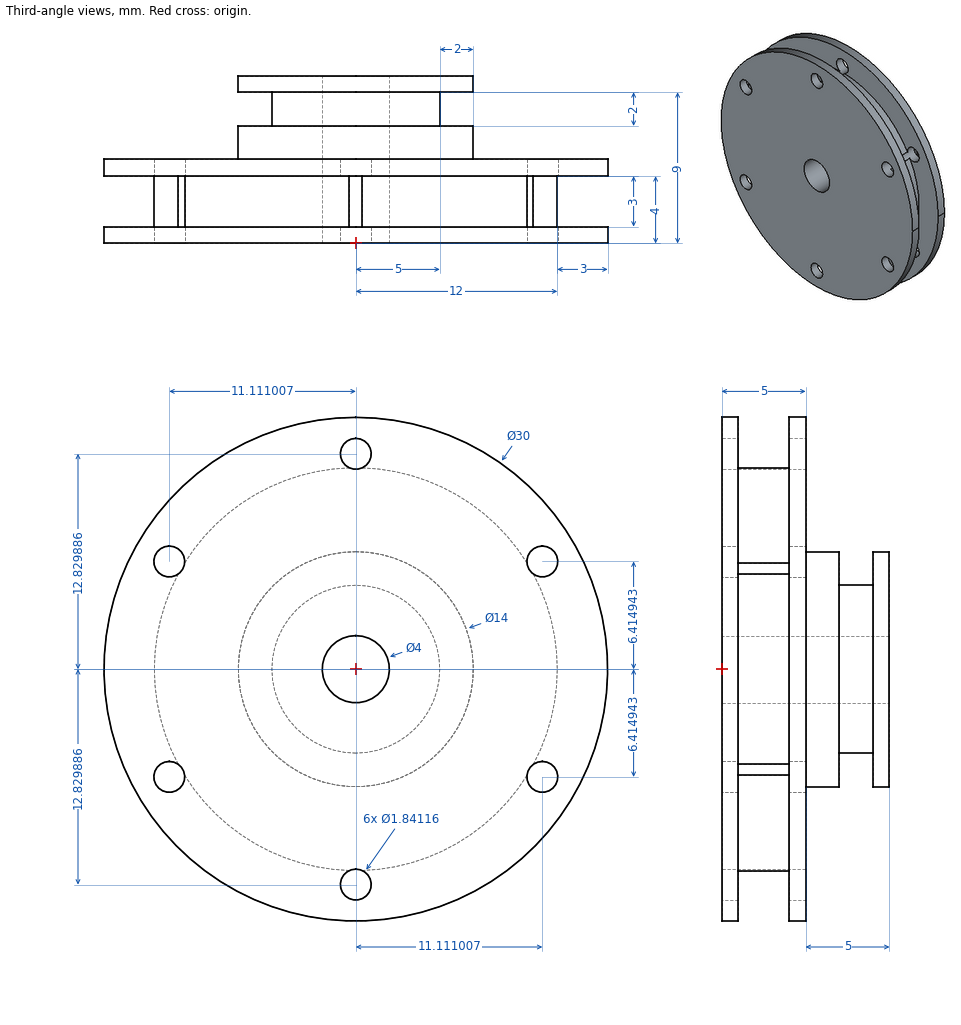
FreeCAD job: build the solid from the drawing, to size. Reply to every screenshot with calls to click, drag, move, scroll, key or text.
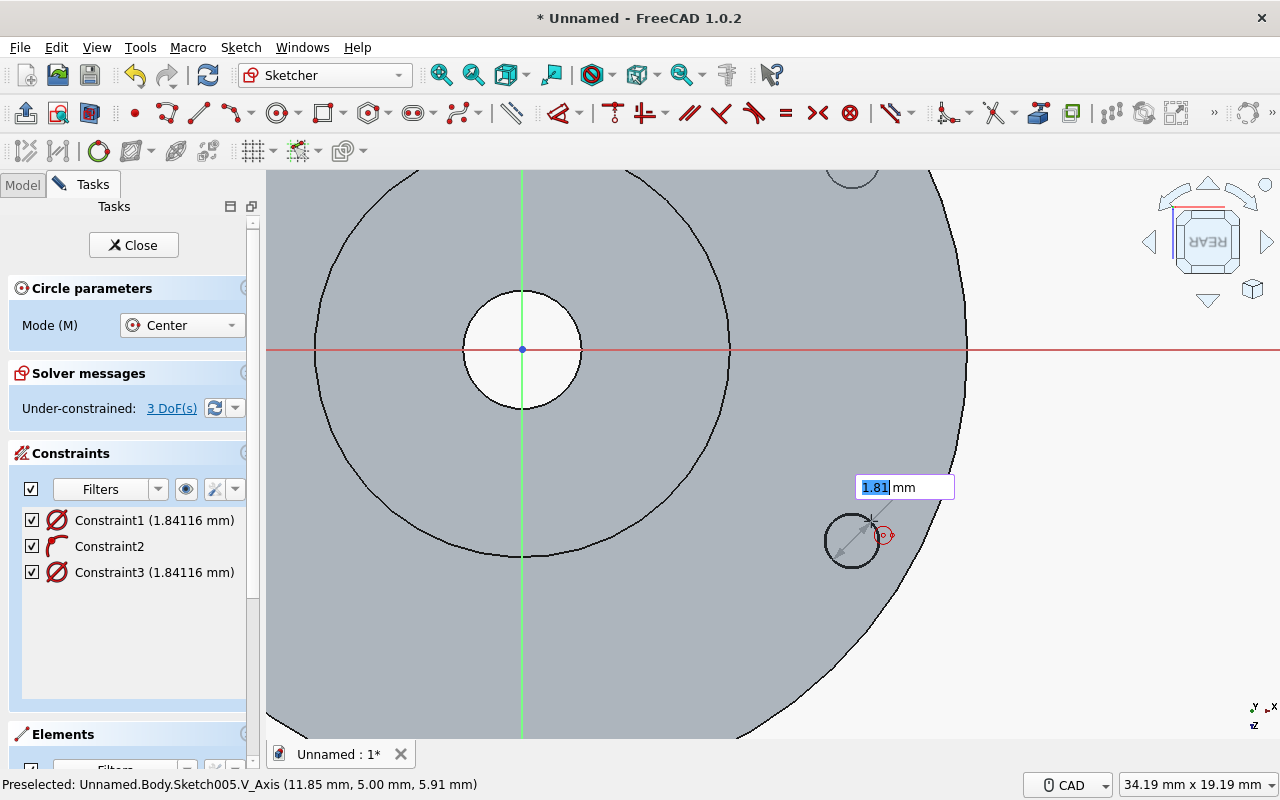
text(1.84116)
key(Return)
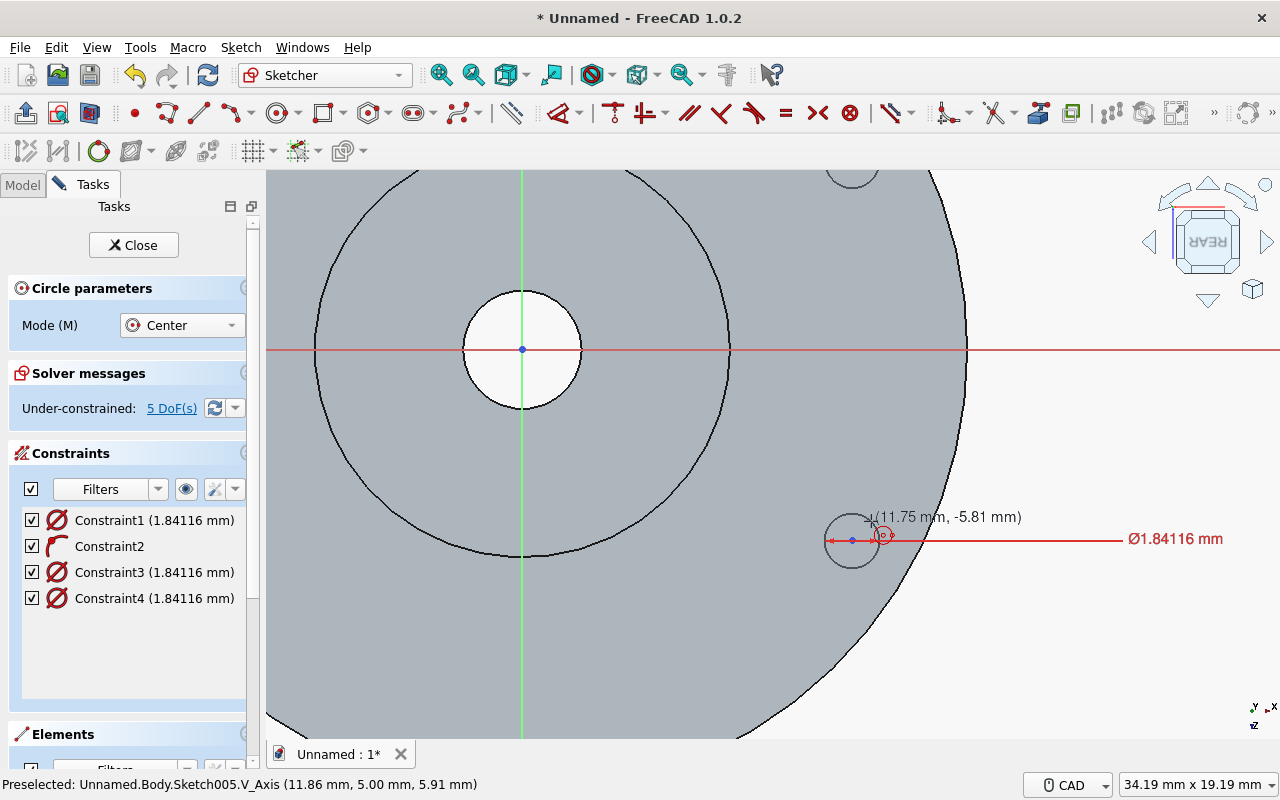
scroll(853, 540, down, 4)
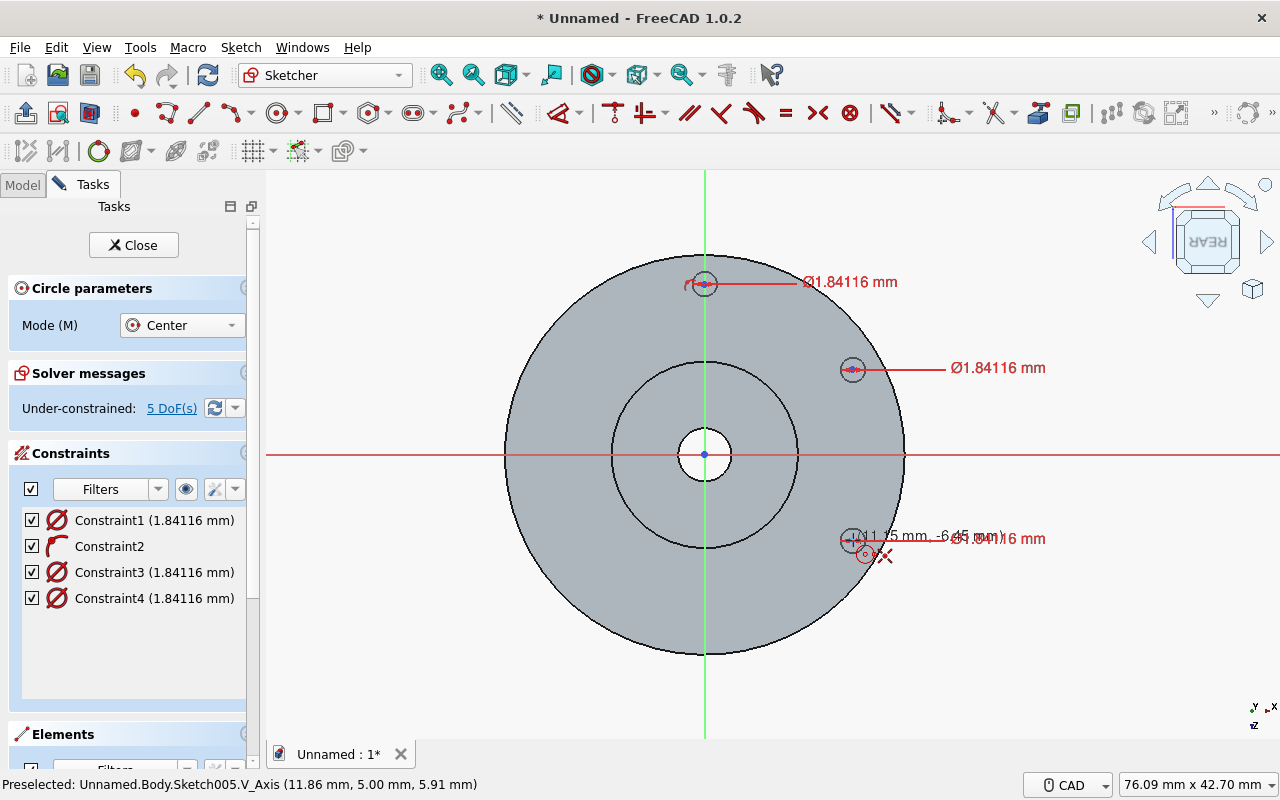
scroll(705, 626, up, 4)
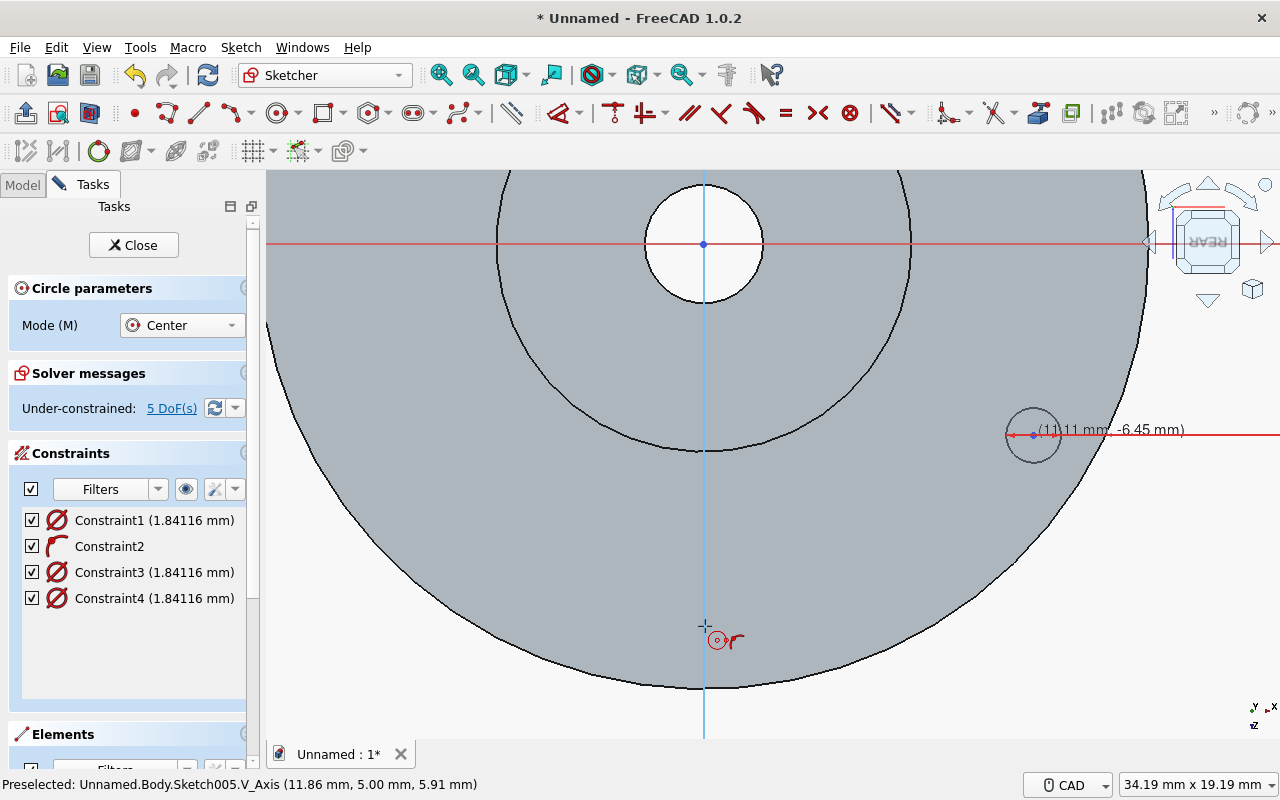
click(704, 625)
move(723, 605)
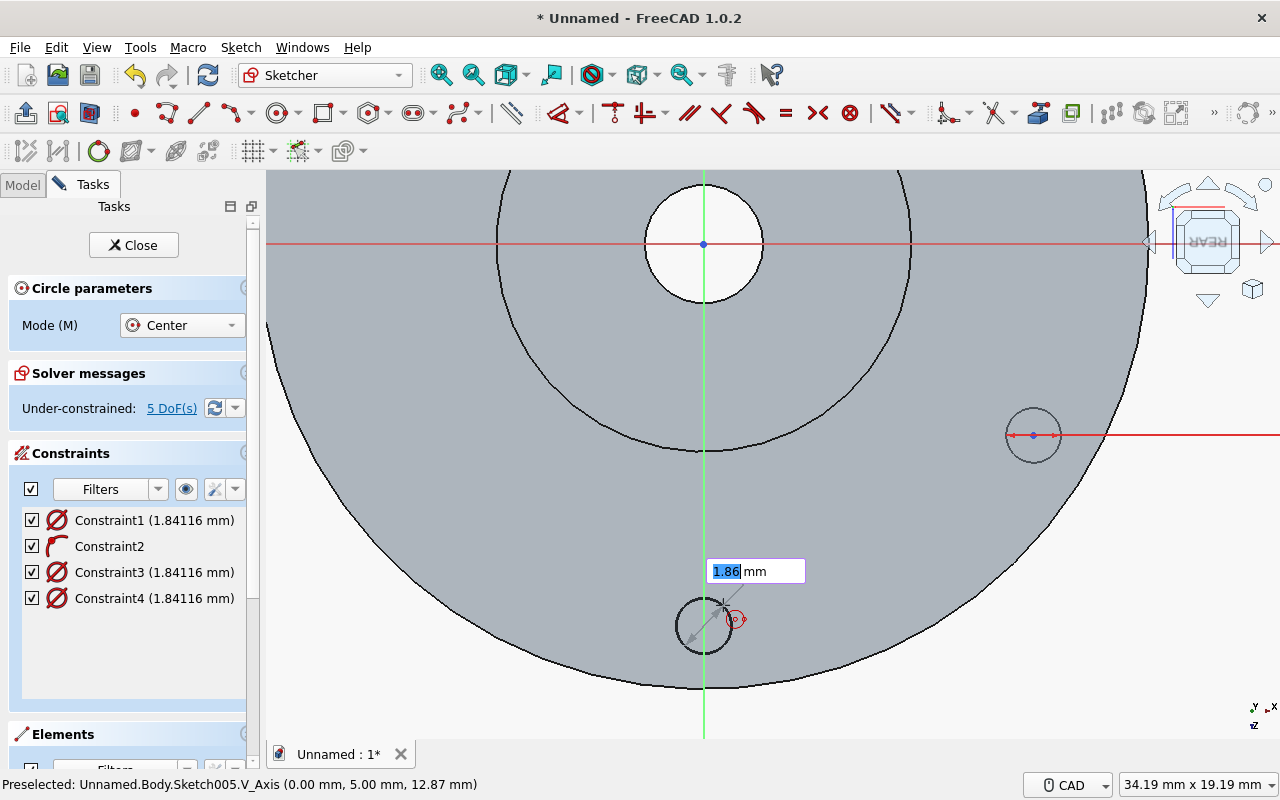
text(1.84116)
key(Return)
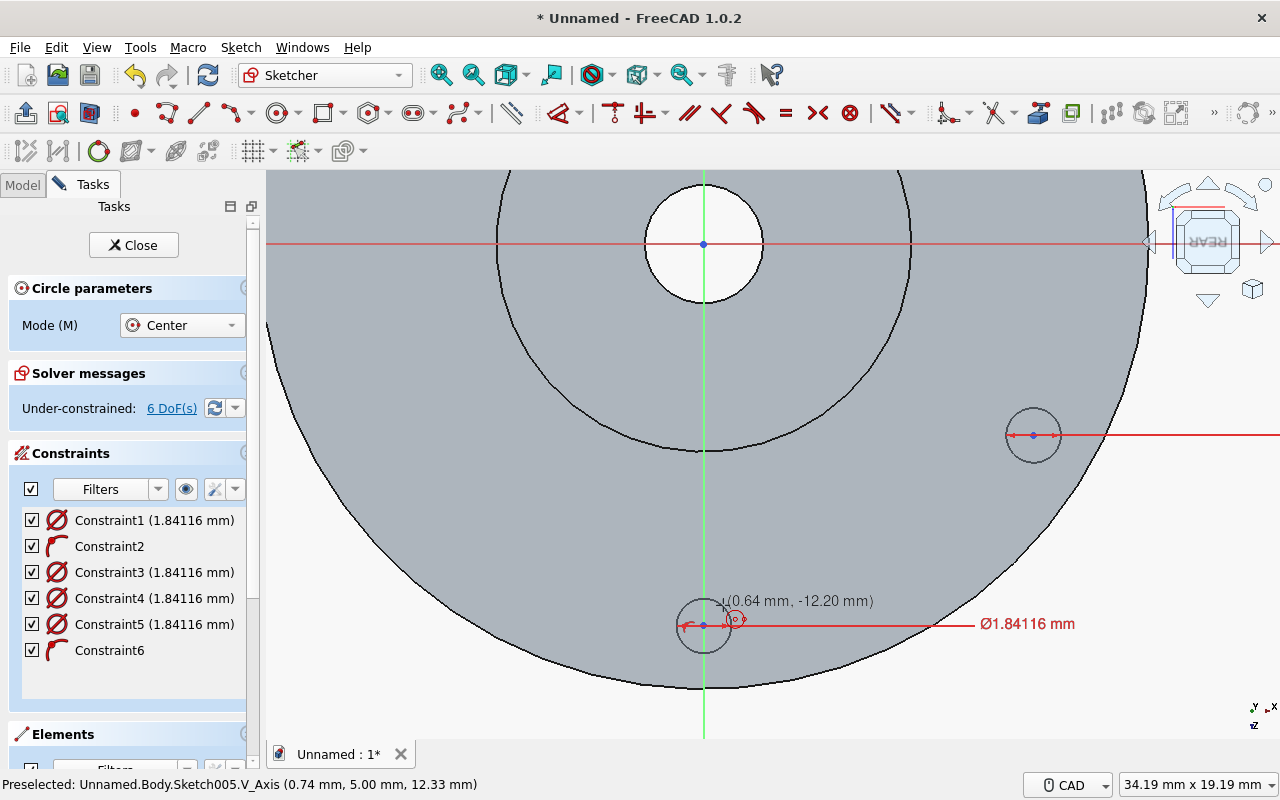
click(374, 434)
move(394, 415)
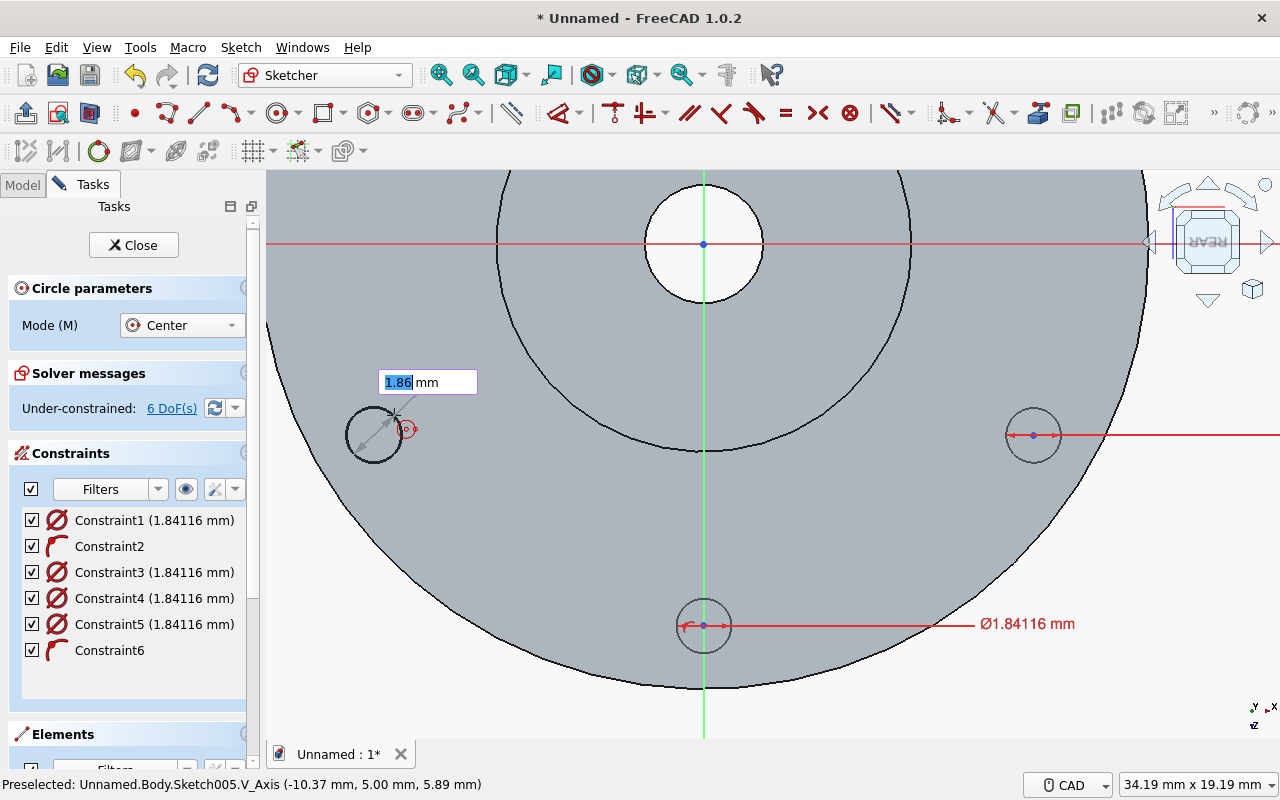
text(1.84116)
key(Return)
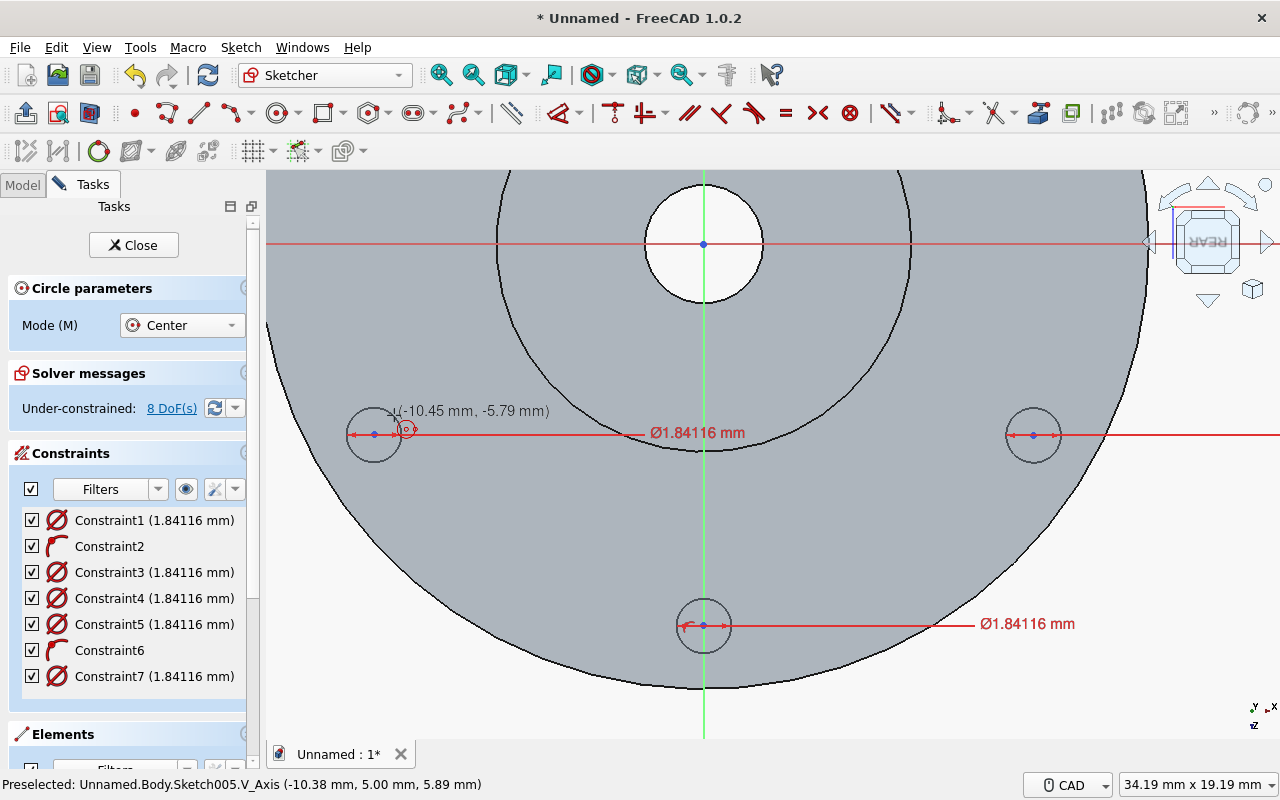
scroll(705, 626, down, 4)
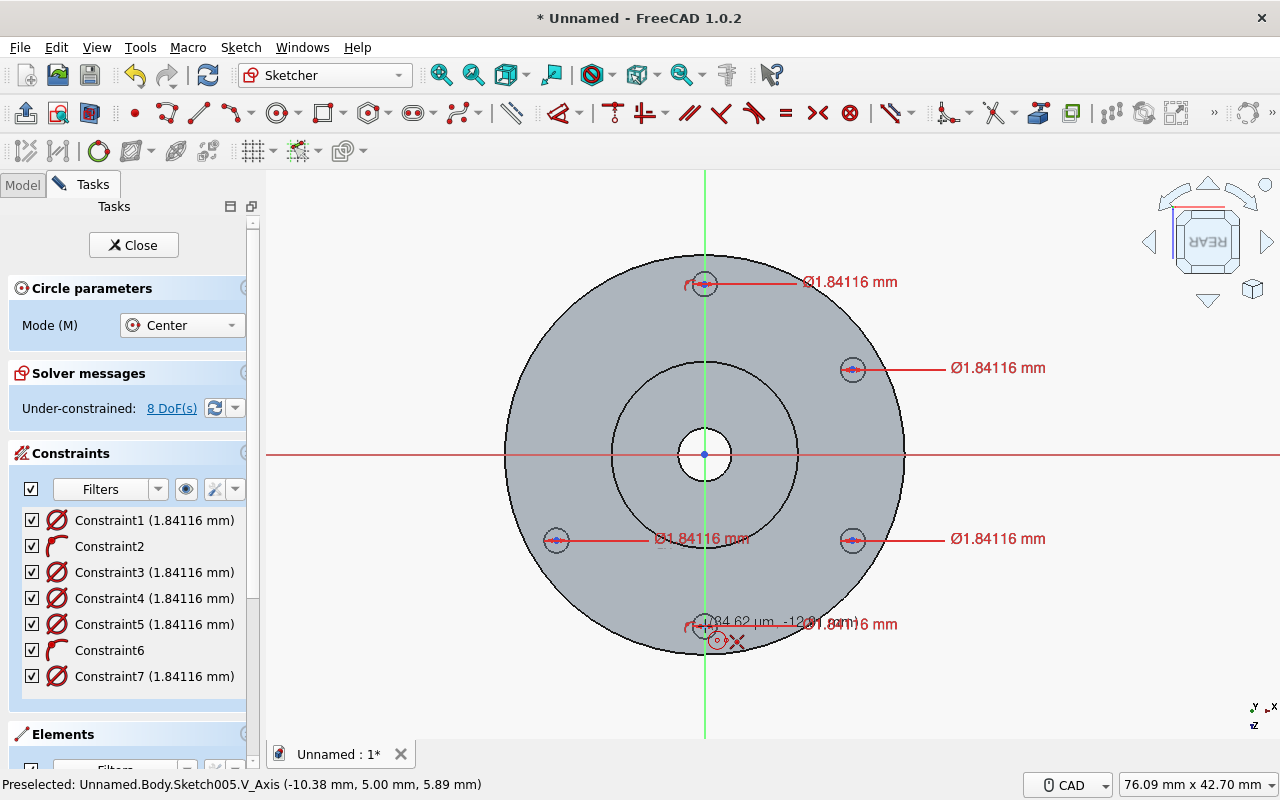
scroll(557, 369, up, 4)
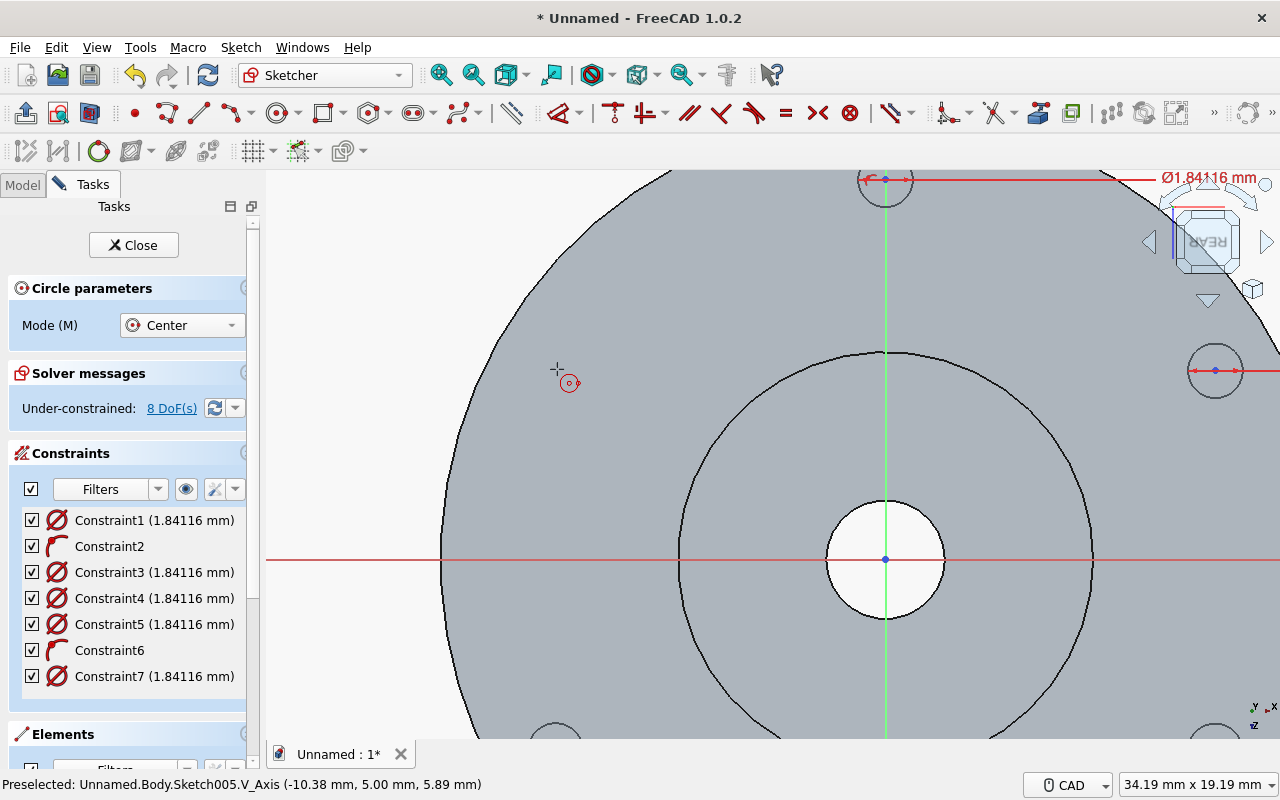
click(556, 369)
move(575, 350)